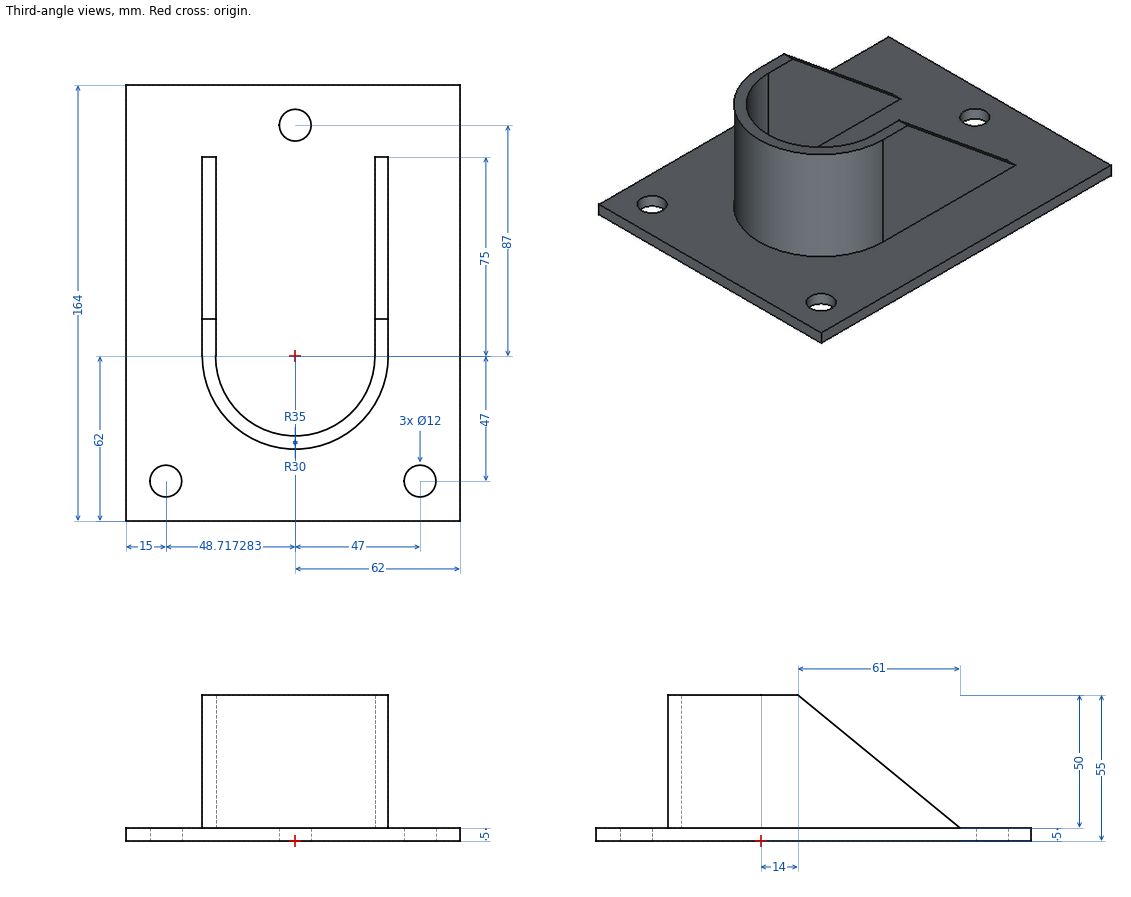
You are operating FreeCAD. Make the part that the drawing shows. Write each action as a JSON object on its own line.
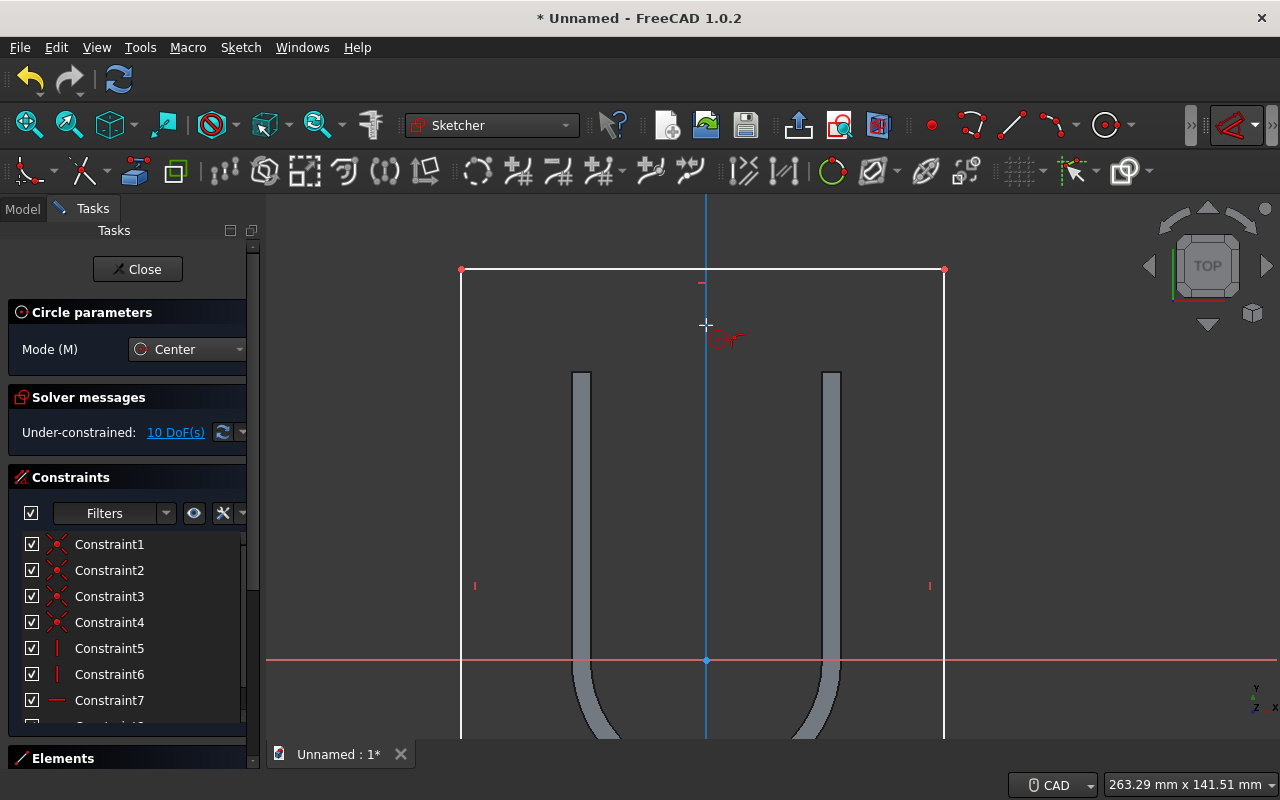
{"action": "left_click", "coordinate": [706, 325]}
{"action": "left_click", "coordinate": [723, 309]}
{"action": "key", "text": "Escape"}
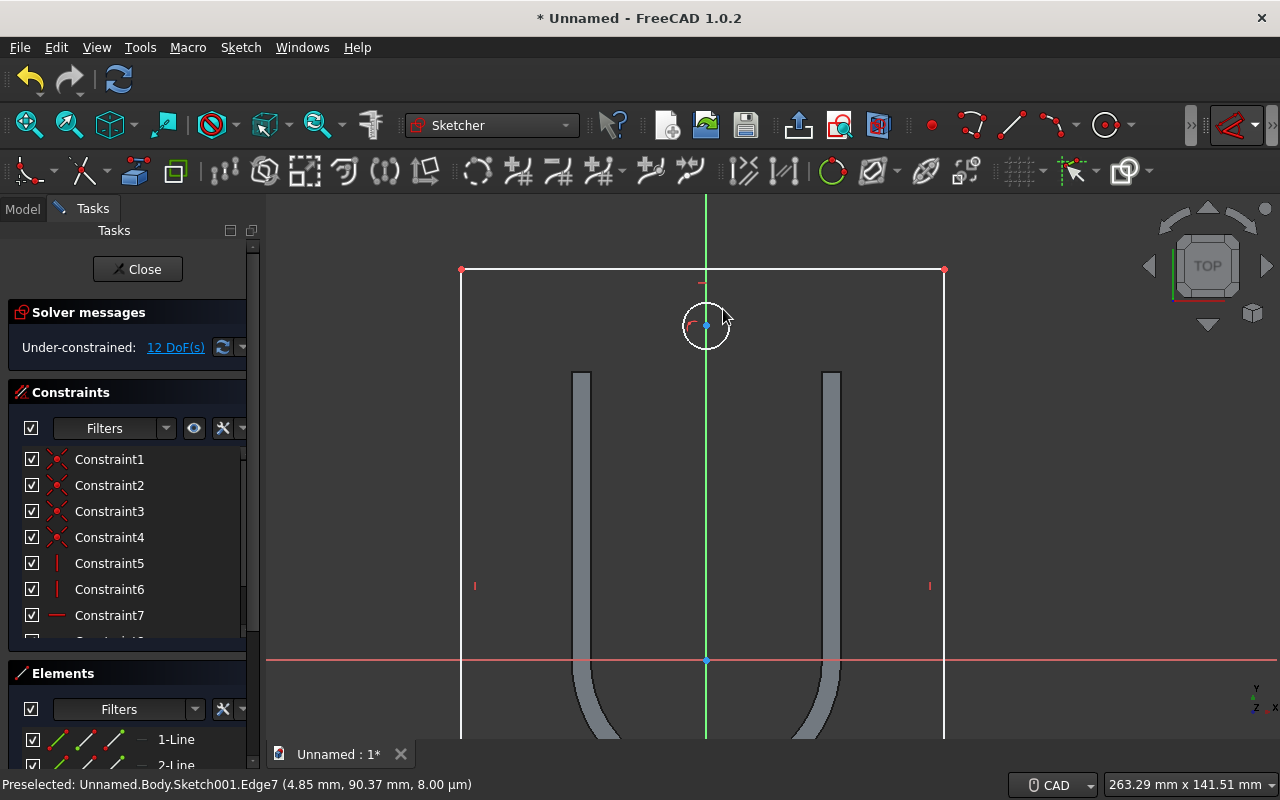
{"action": "scroll", "coordinate": [706, 324], "scroll_direction": "down", "scroll_amount": 3}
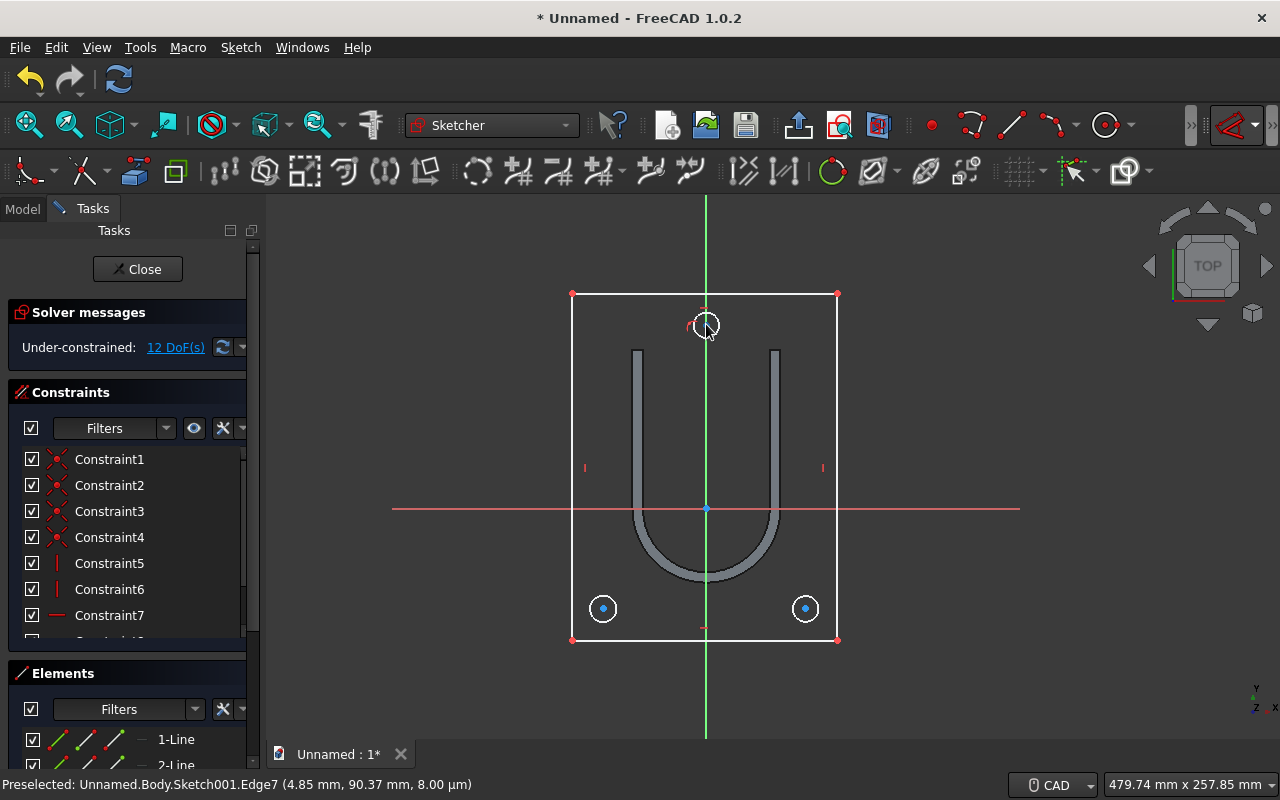
{"action": "left_click", "coordinate": [815, 600]}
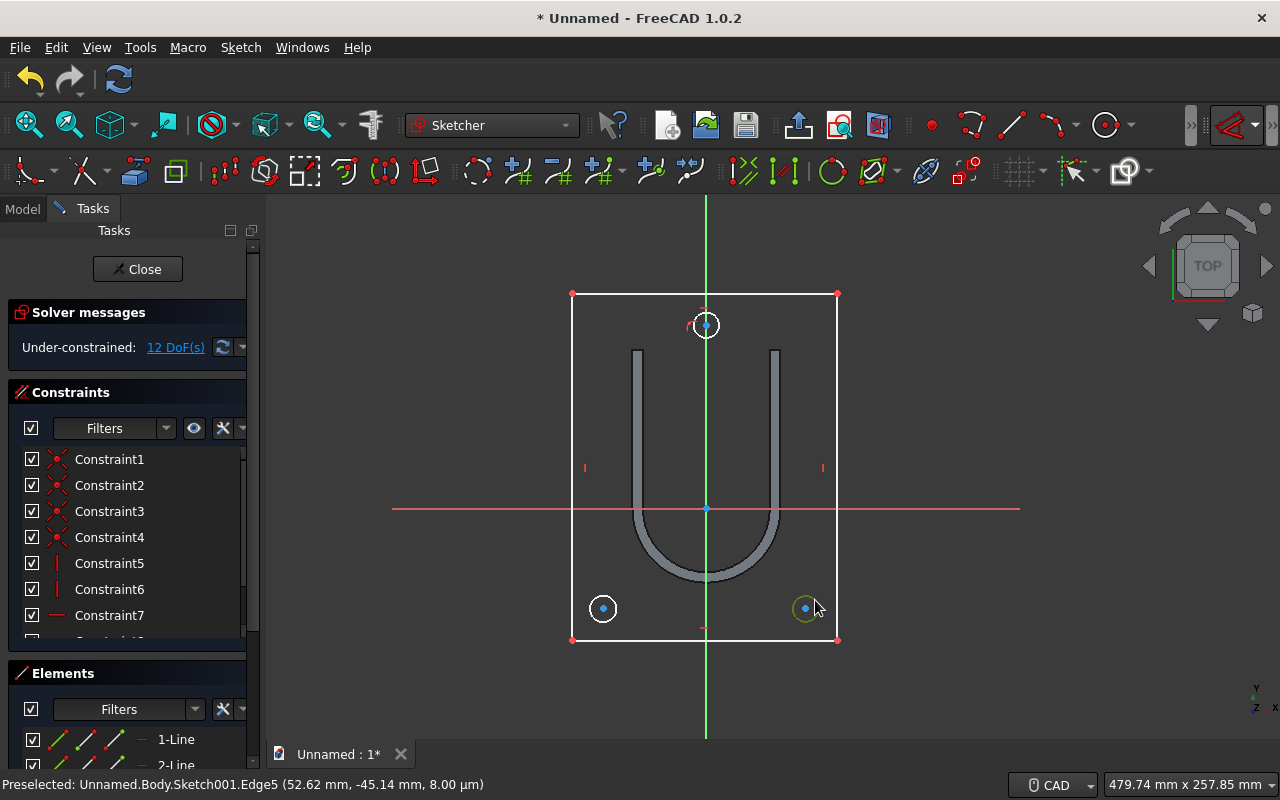
{"action": "left_click", "coordinate": [612, 600]}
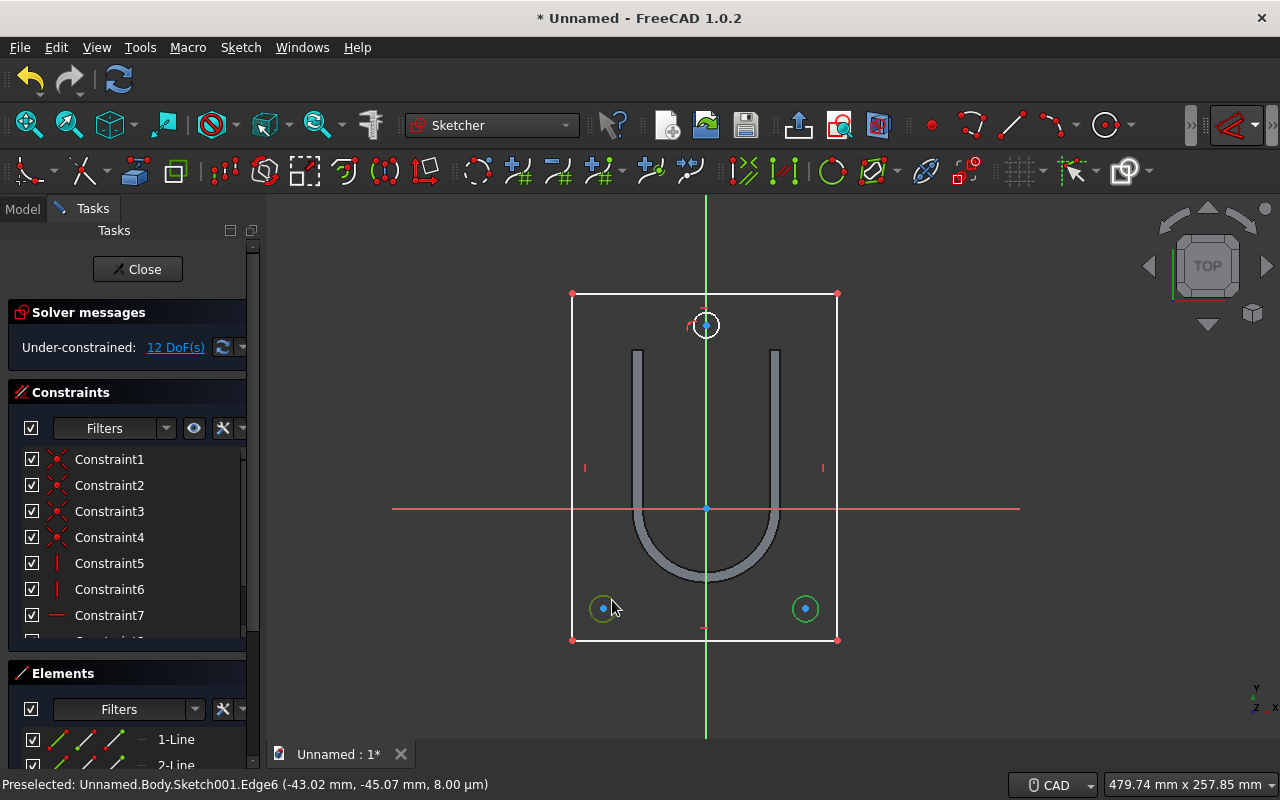
{"action": "left_click", "coordinate": [707, 313]}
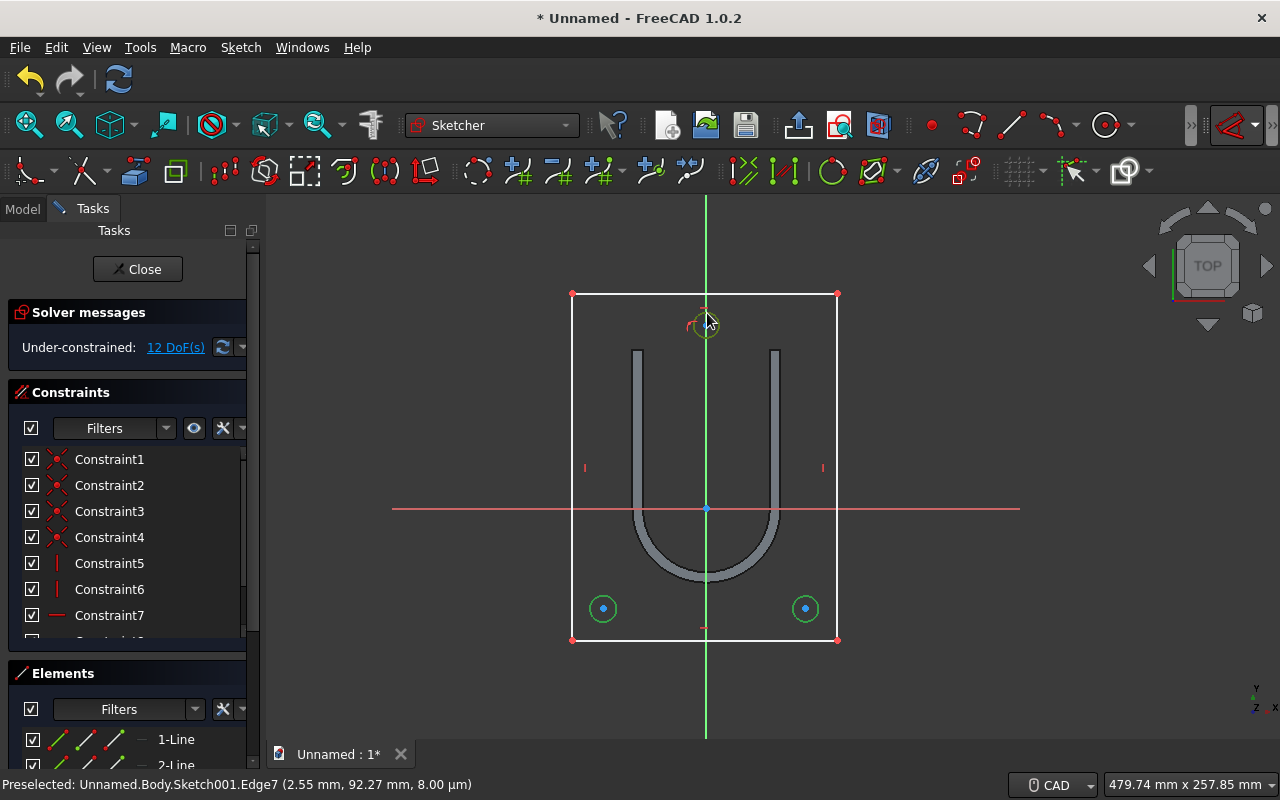
{"action": "key", "text": "e"}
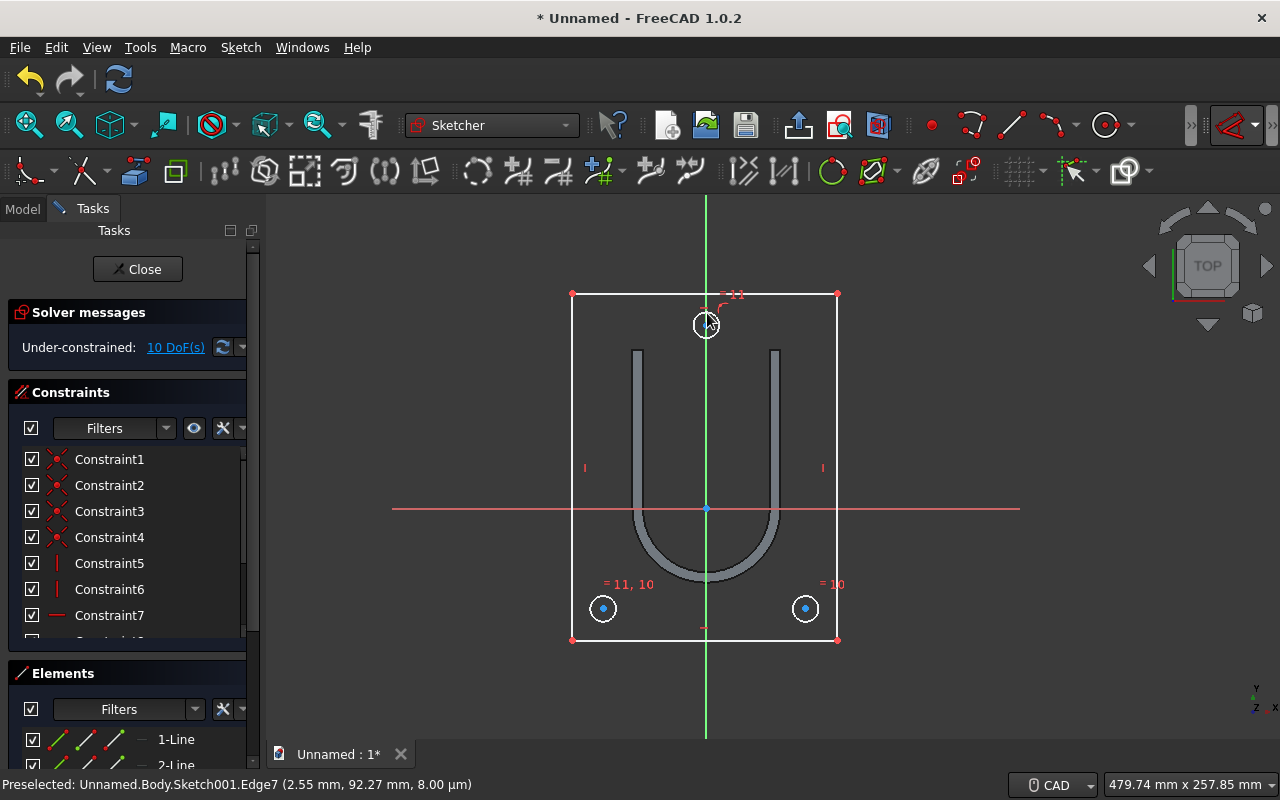
{"action": "left_click", "coordinate": [806, 609]}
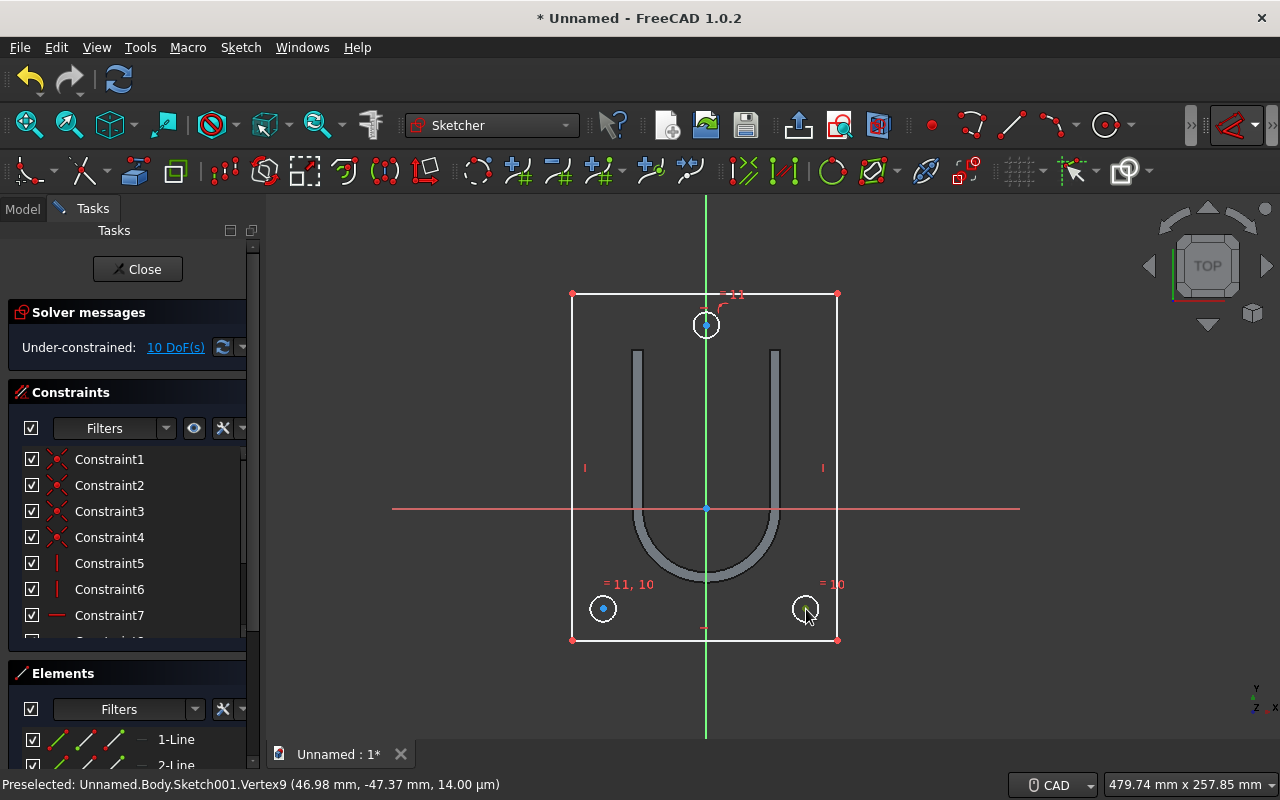
{"action": "left_click", "coordinate": [603, 609]}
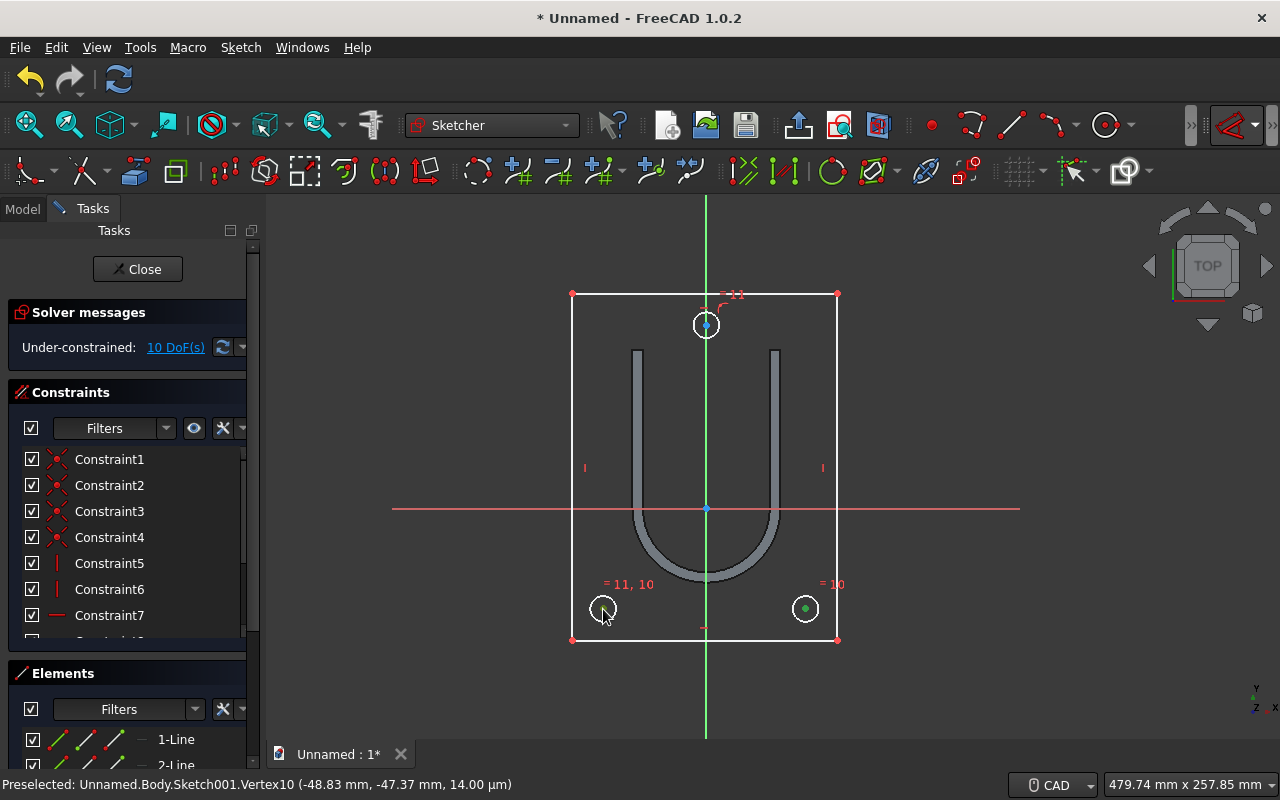
{"action": "key", "text": "h"}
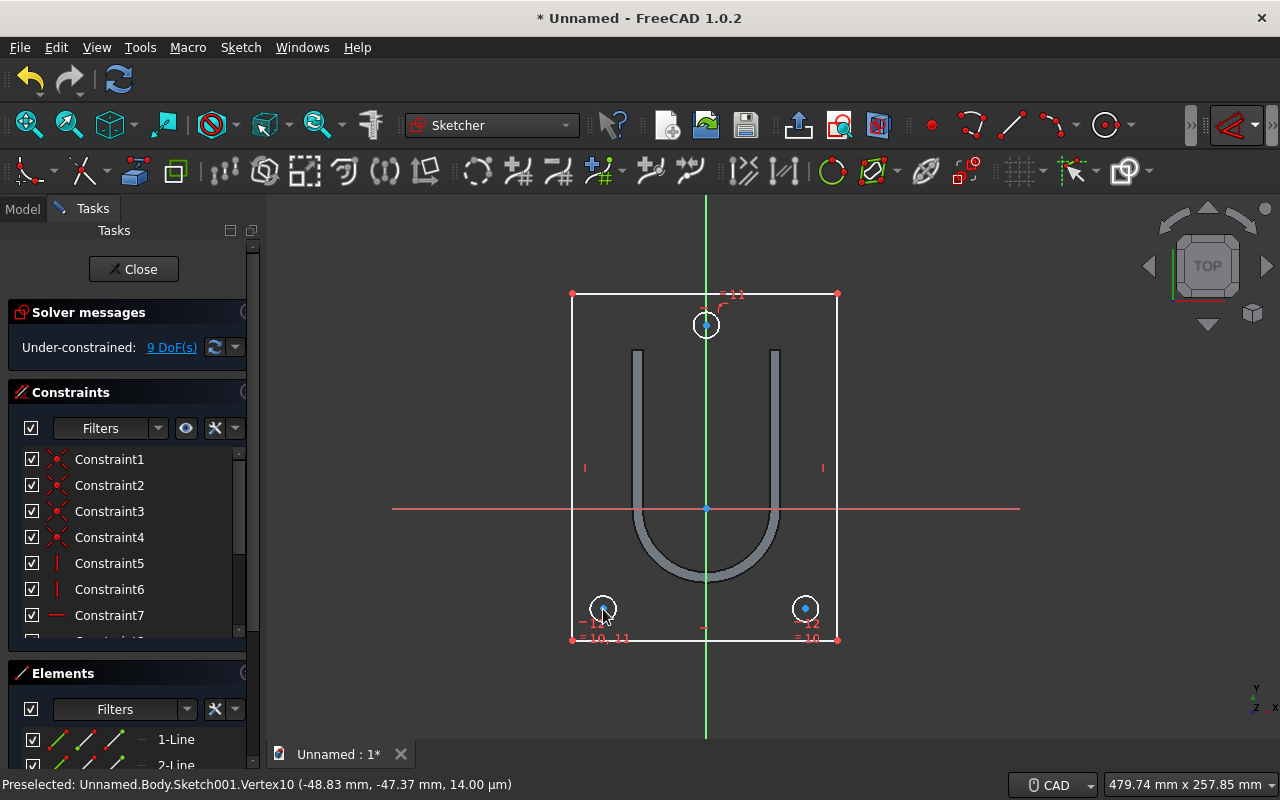
{"action": "scroll", "coordinate": [815, 600], "scroll_direction": "up", "scroll_amount": 3}